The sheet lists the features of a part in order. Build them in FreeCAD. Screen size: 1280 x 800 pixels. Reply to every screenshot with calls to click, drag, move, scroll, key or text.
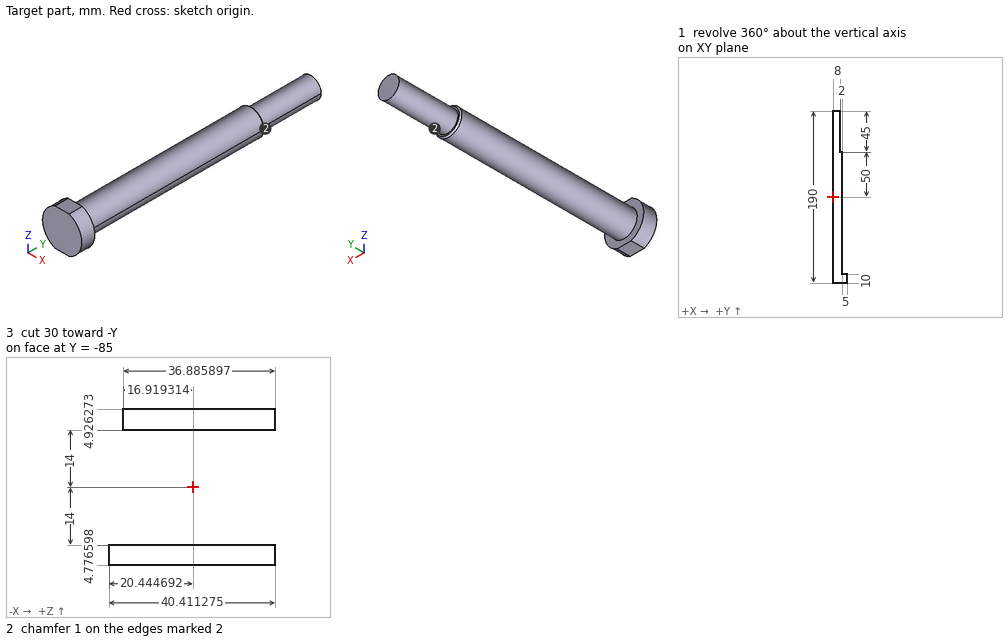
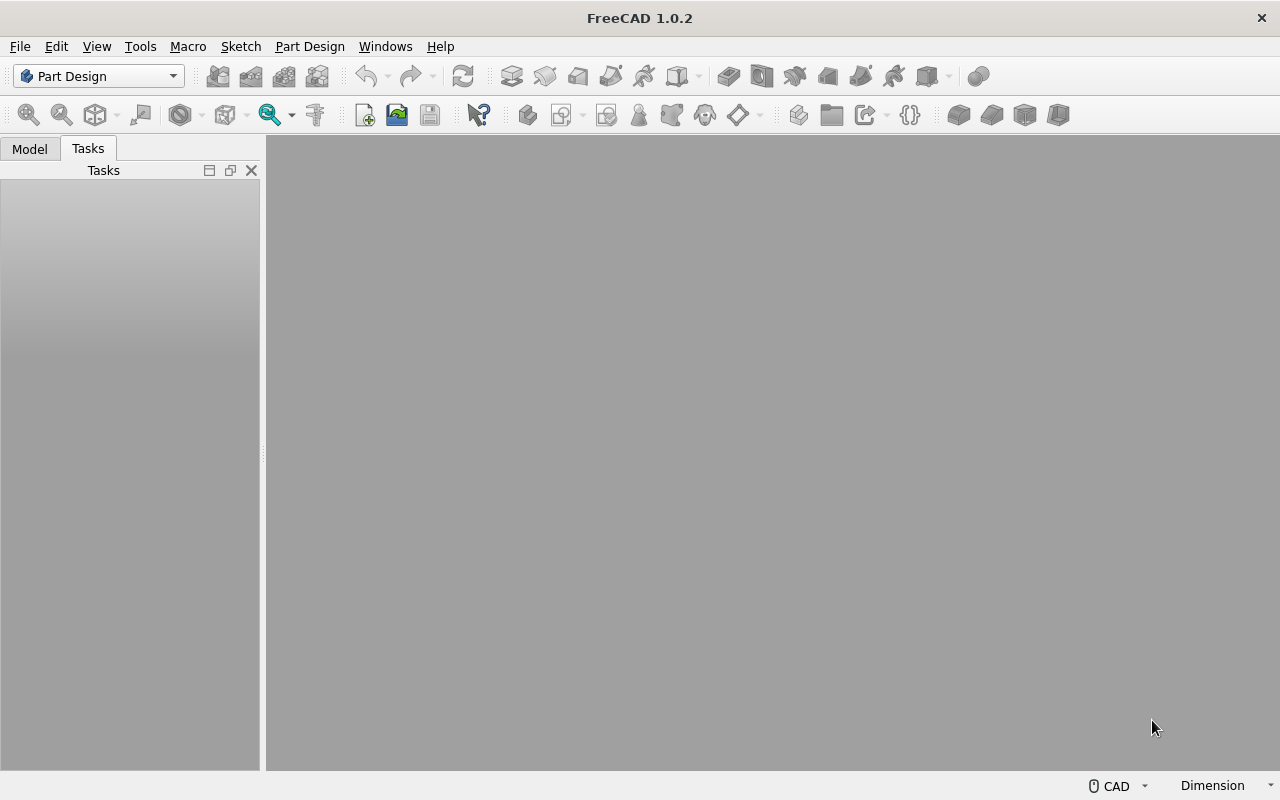
click(364, 116)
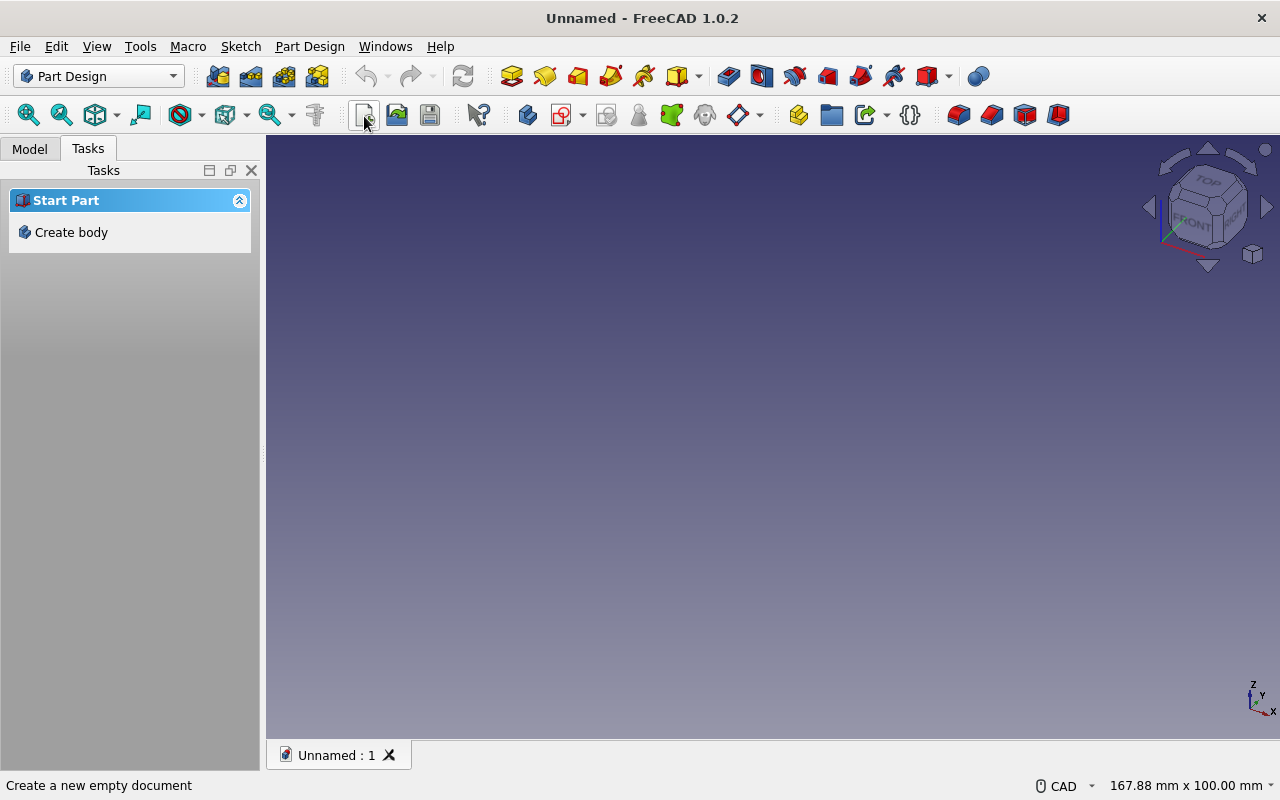
click(560, 116)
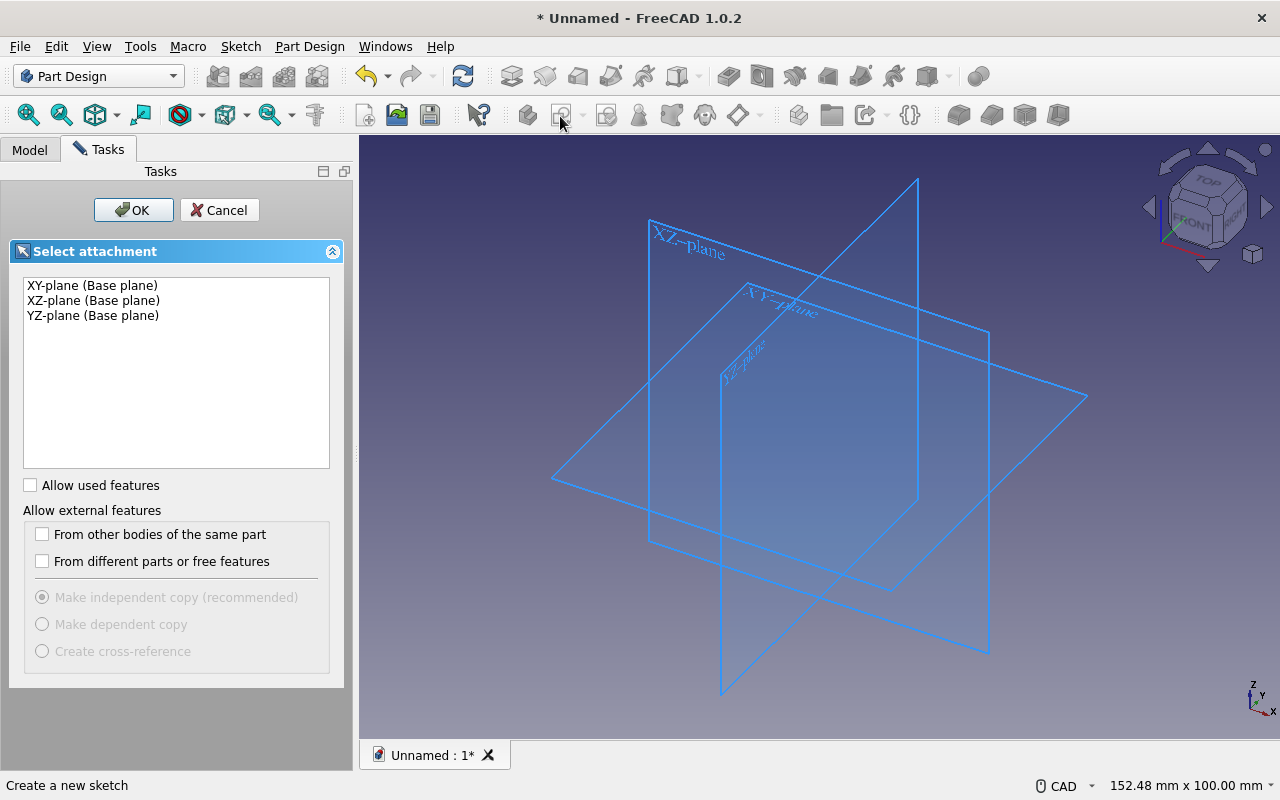
click(84, 286)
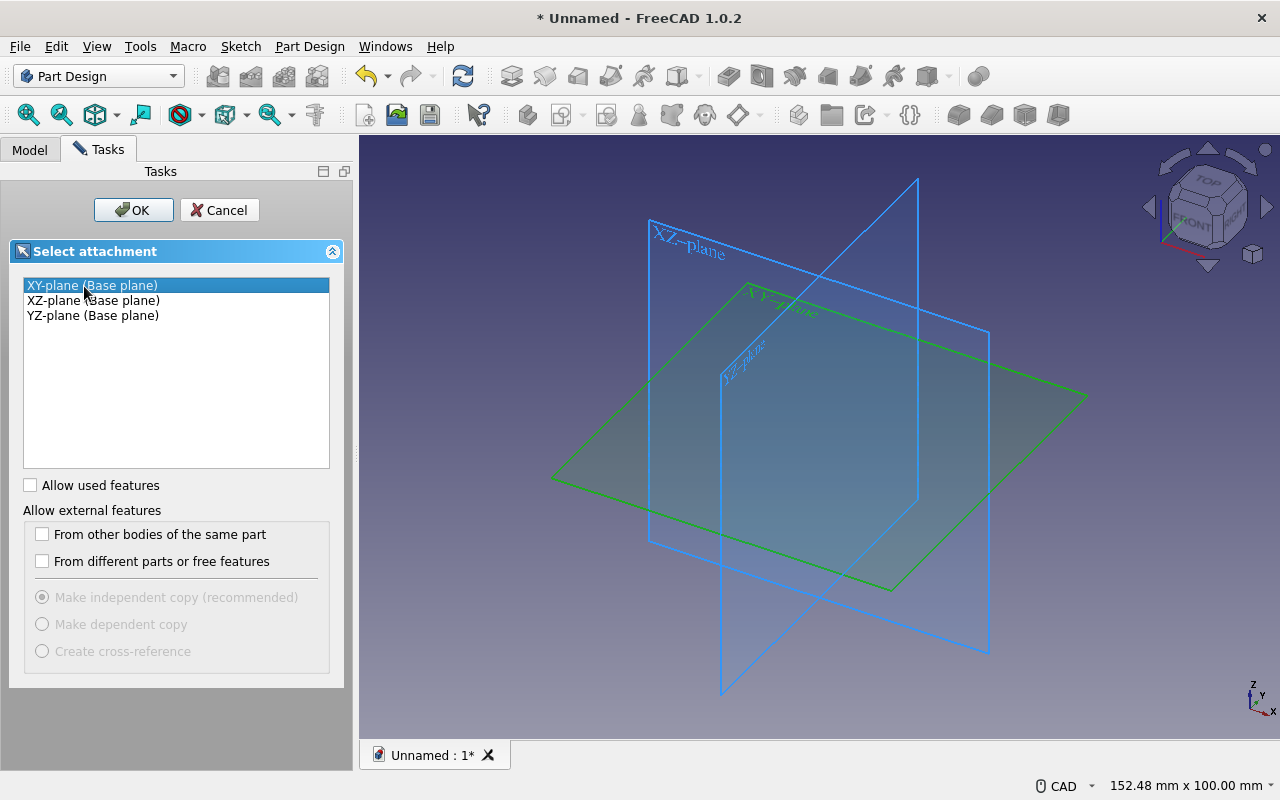
click(134, 210)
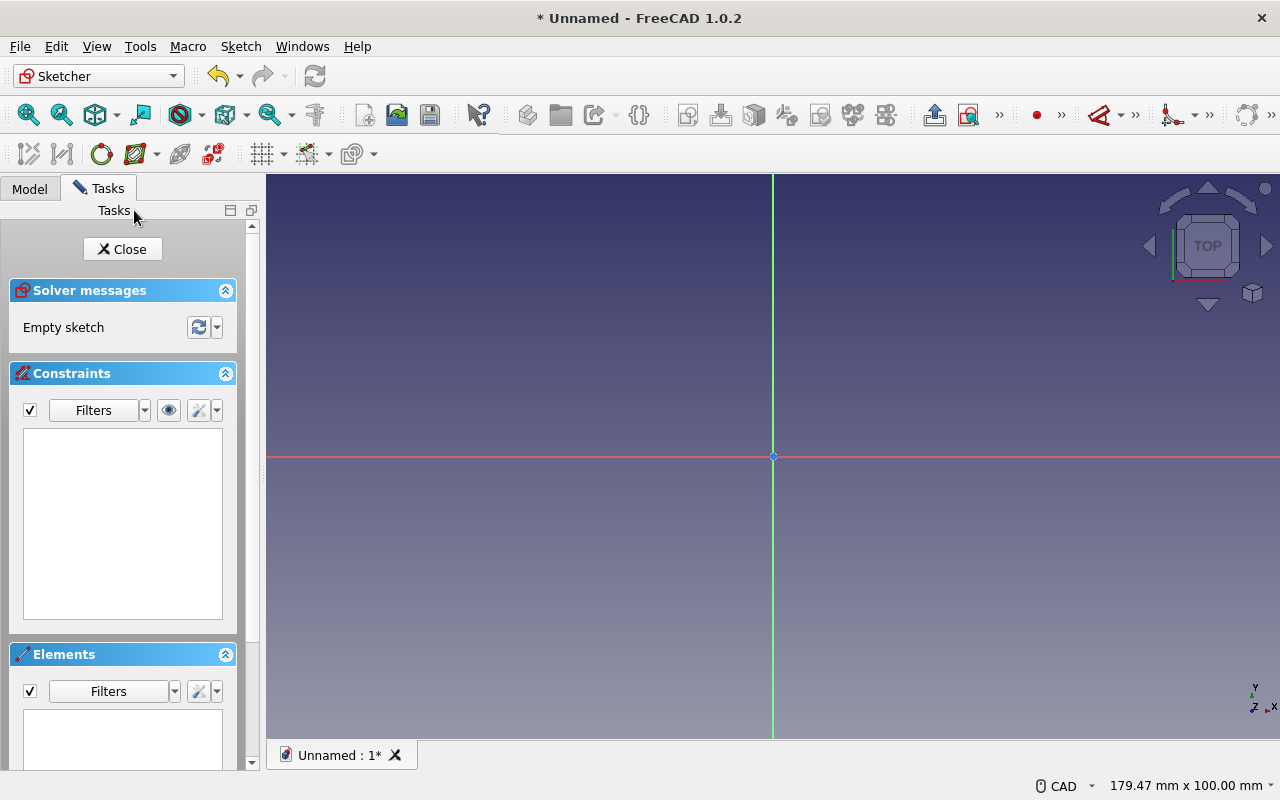
scroll(640, 456, down, 5)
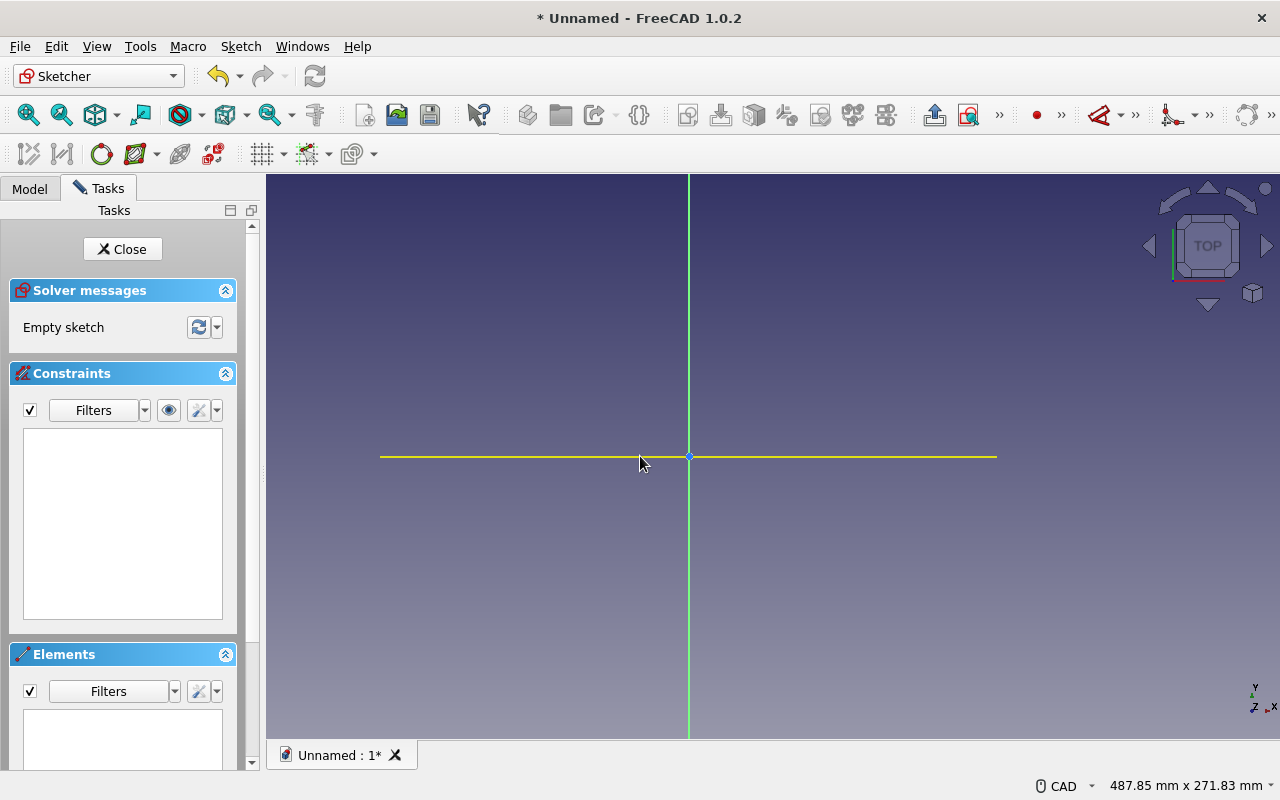
key(g)
key(m)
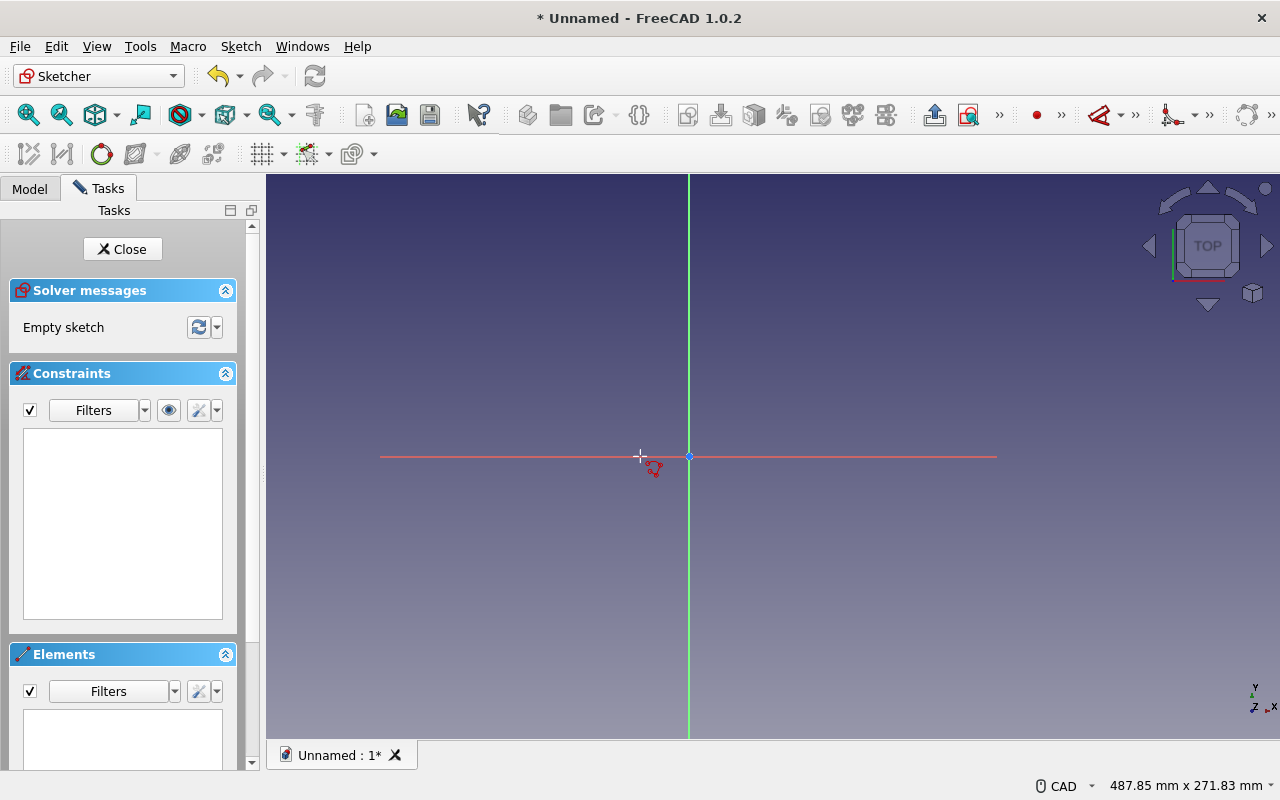
click(706, 353)
click(706, 259)
click(689, 259)
click(698, 654)
click(720, 654)
click(720, 633)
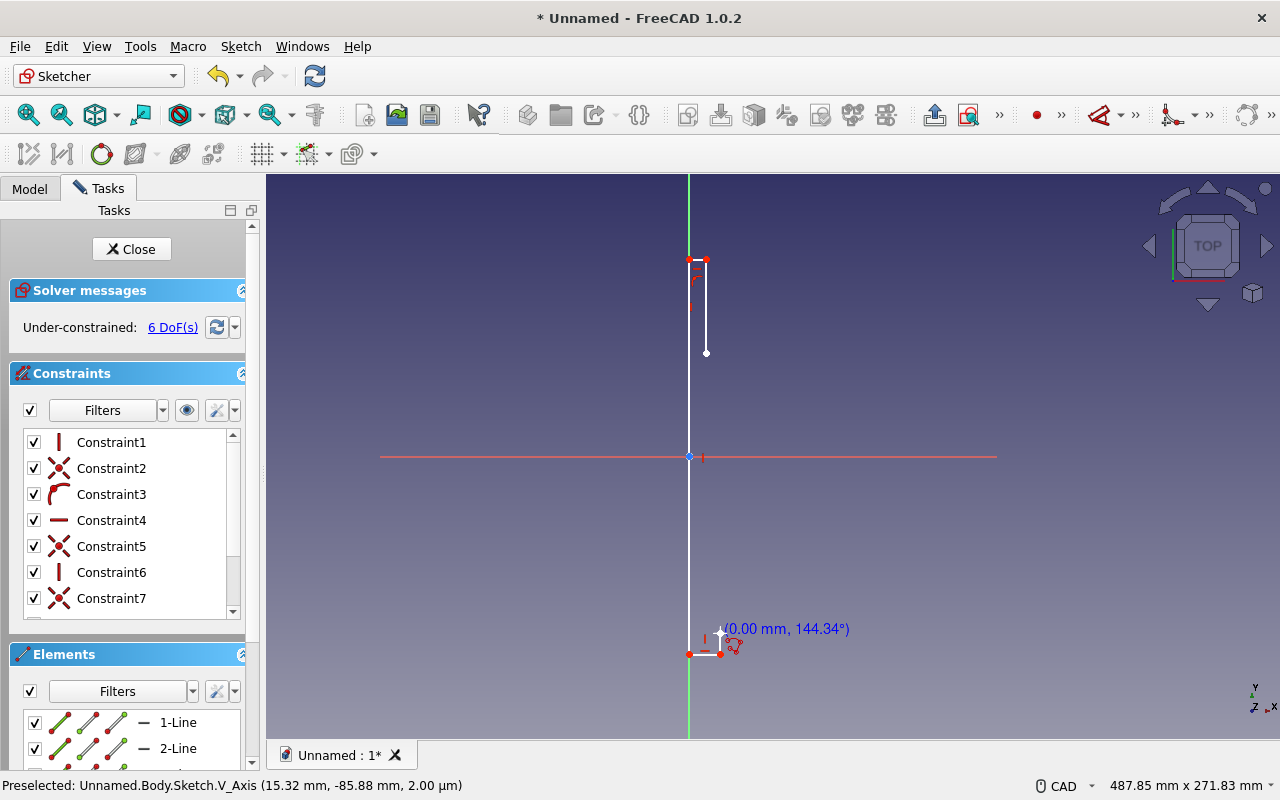
scroll(710, 633, up, 3)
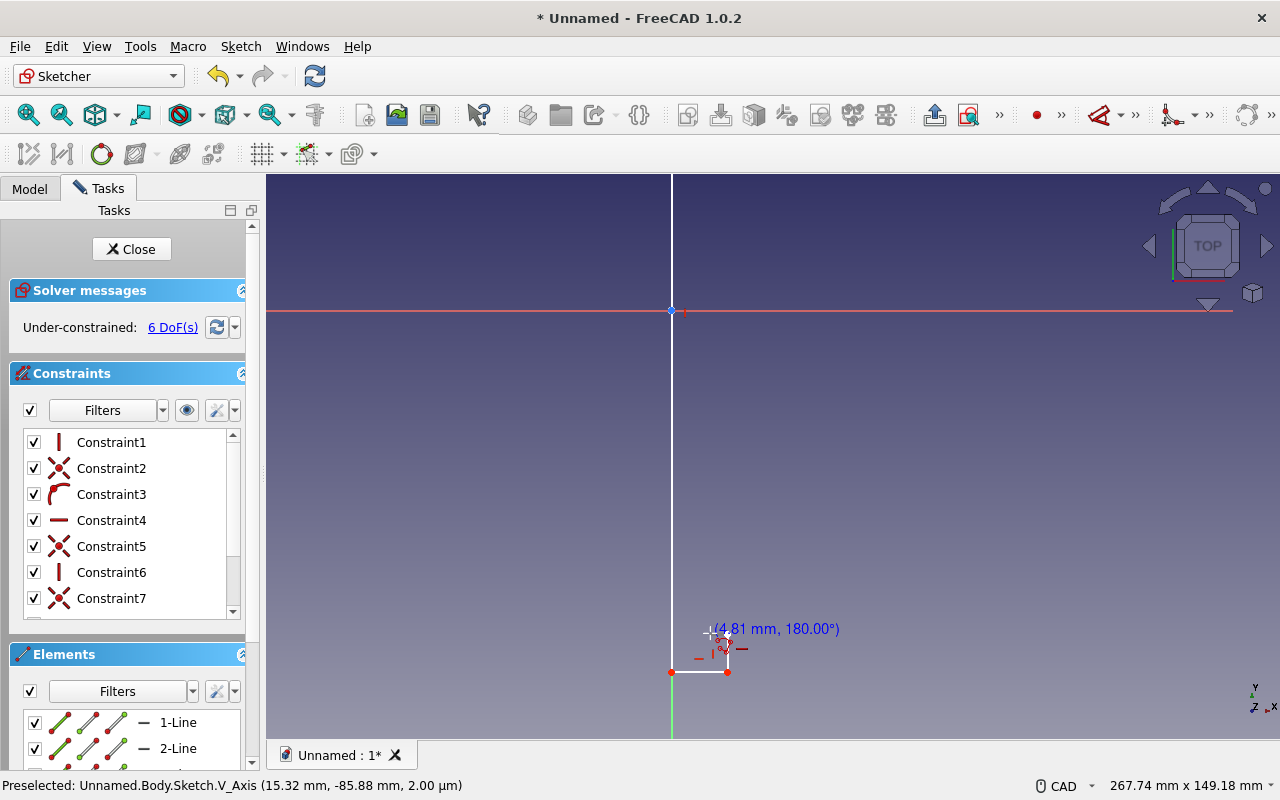
click(710, 632)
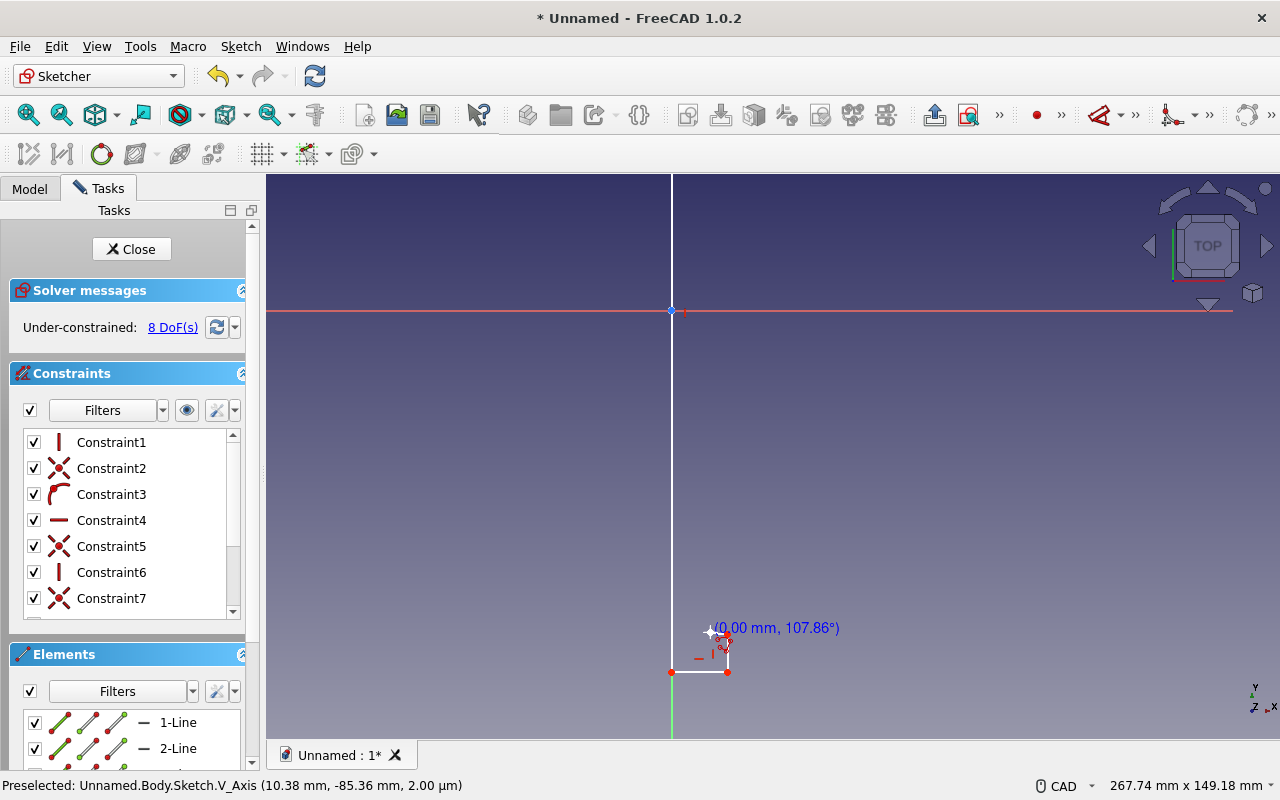
scroll(710, 634, down, 3)